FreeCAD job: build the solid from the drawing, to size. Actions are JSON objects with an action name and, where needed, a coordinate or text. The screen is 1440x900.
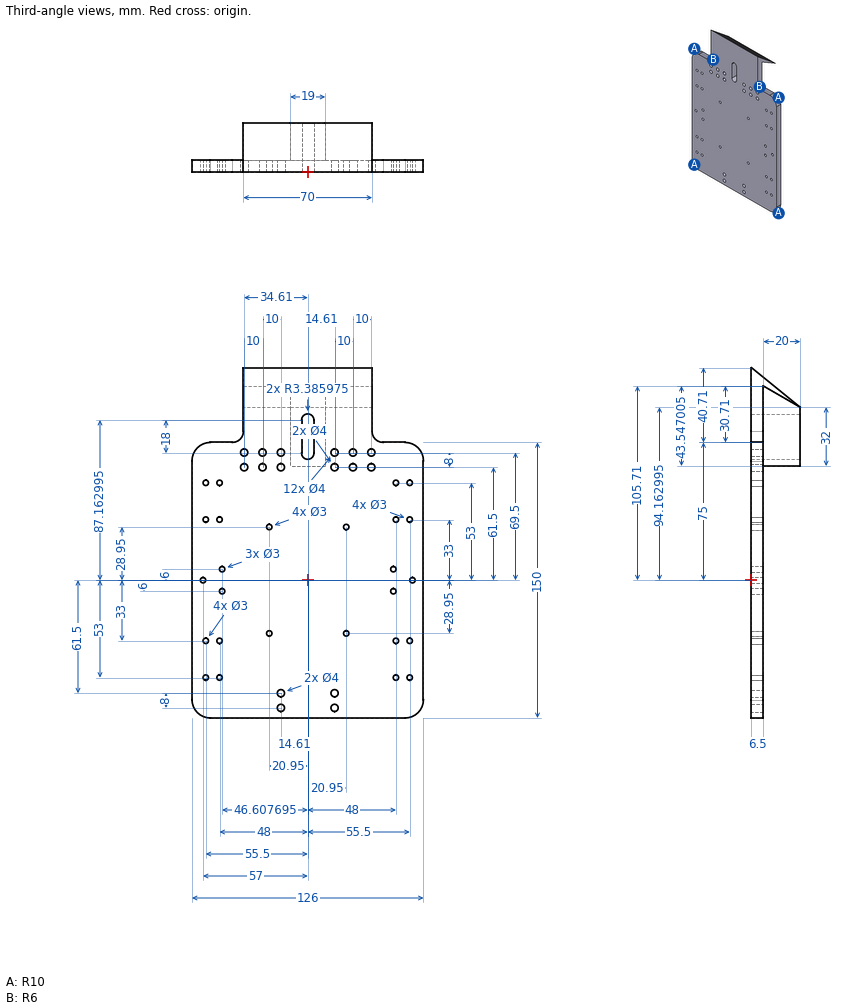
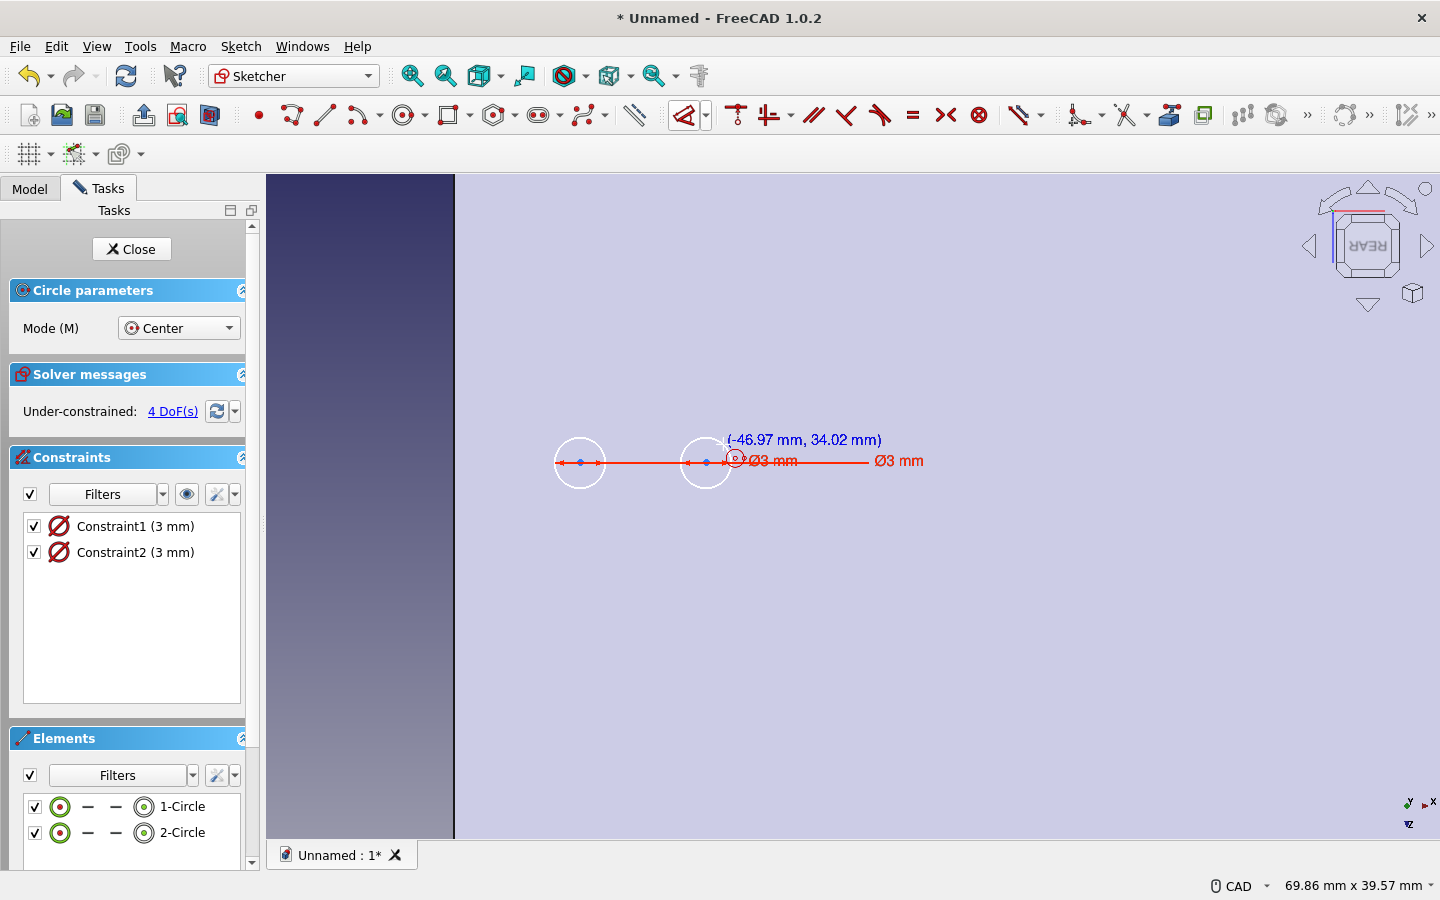
{"action": "scroll", "coordinate": [581, 464], "scroll_direction": "down", "scroll_amount": 4}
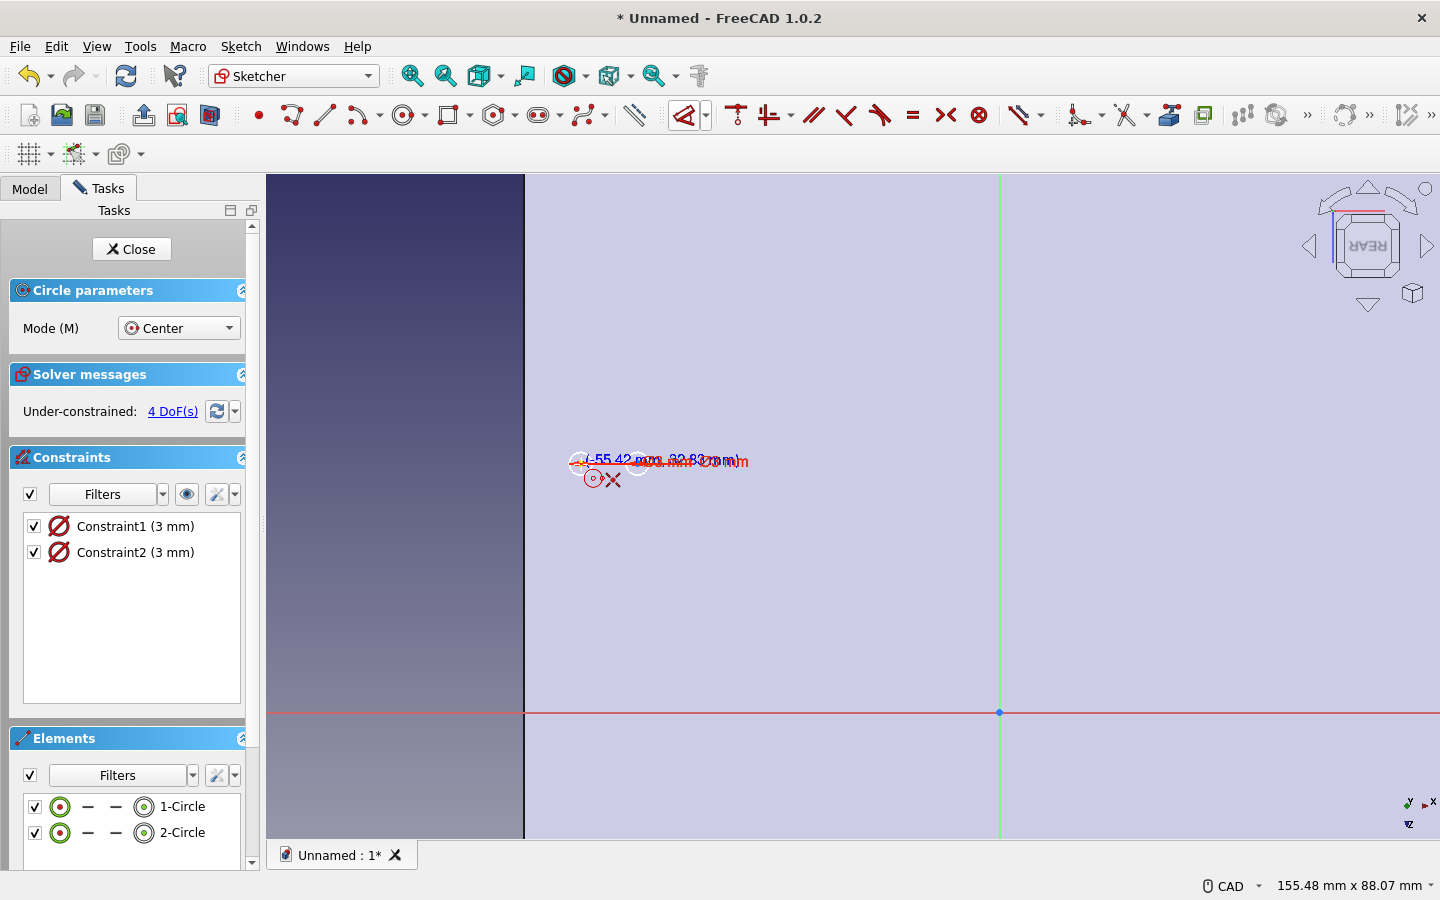
{"action": "scroll", "coordinate": [637, 312], "scroll_direction": "up", "scroll_amount": 4}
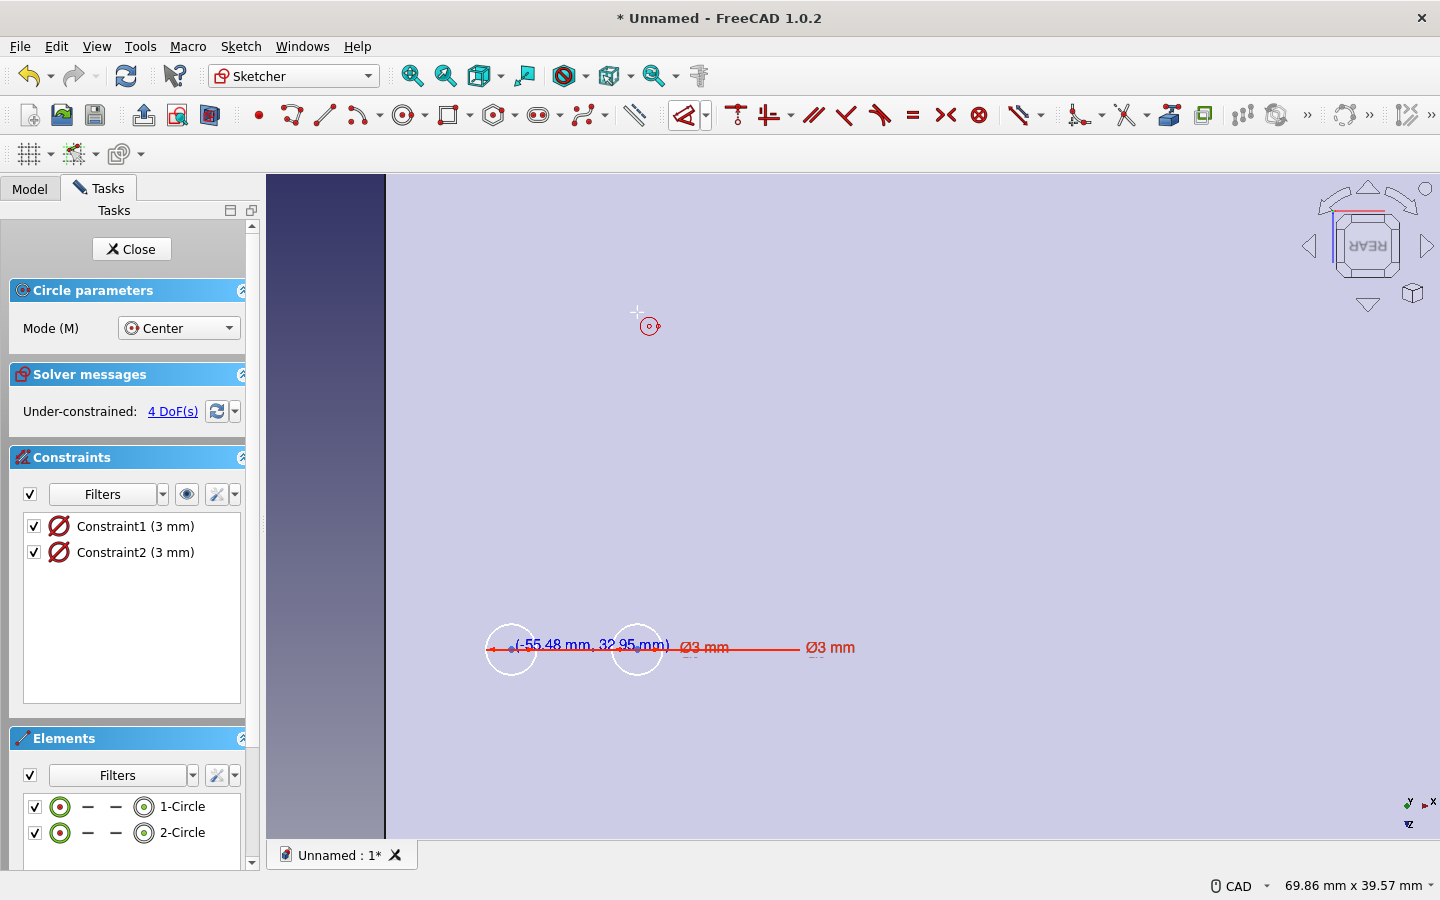
{"action": "left_click", "coordinate": [637, 313]}
{"action": "mouse_move", "coordinate": [655, 295]}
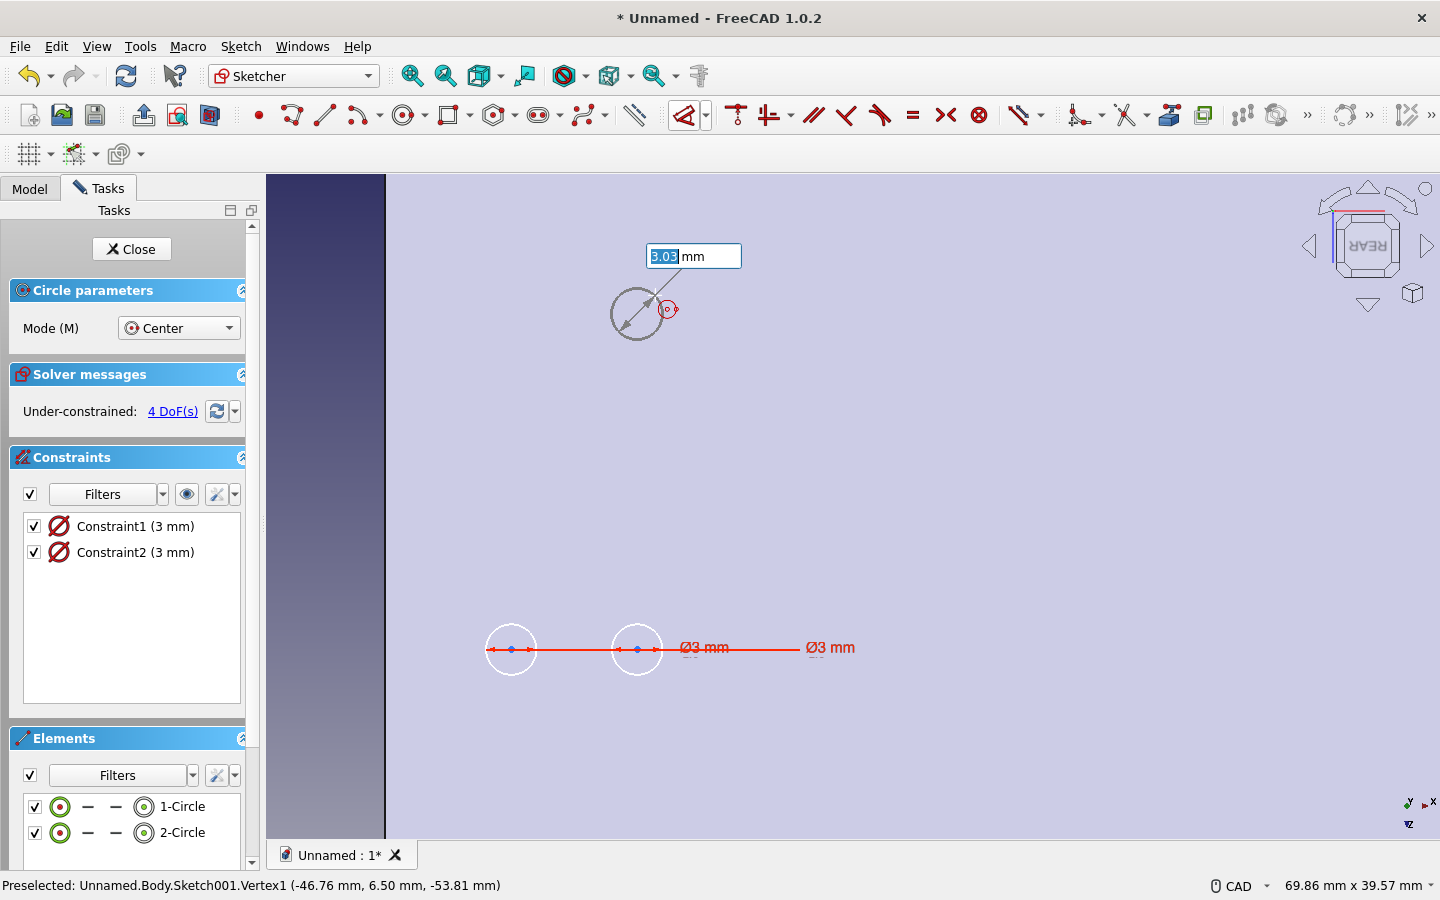
{"action": "type", "text": "3"}
{"action": "key", "text": "Return"}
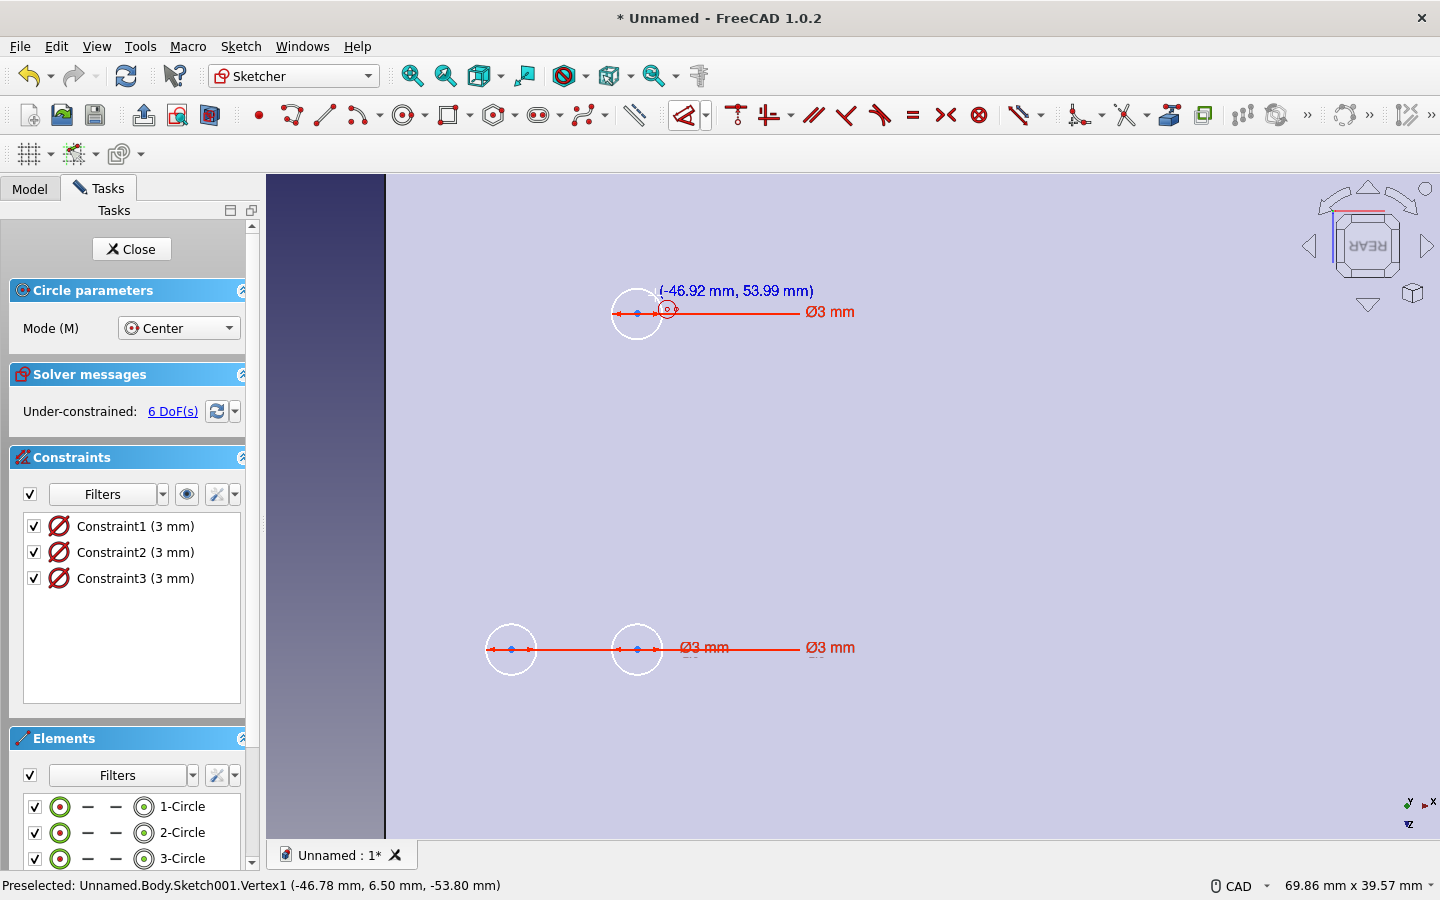
{"action": "left_click", "coordinate": [511, 313]}
{"action": "mouse_move", "coordinate": [529, 295]}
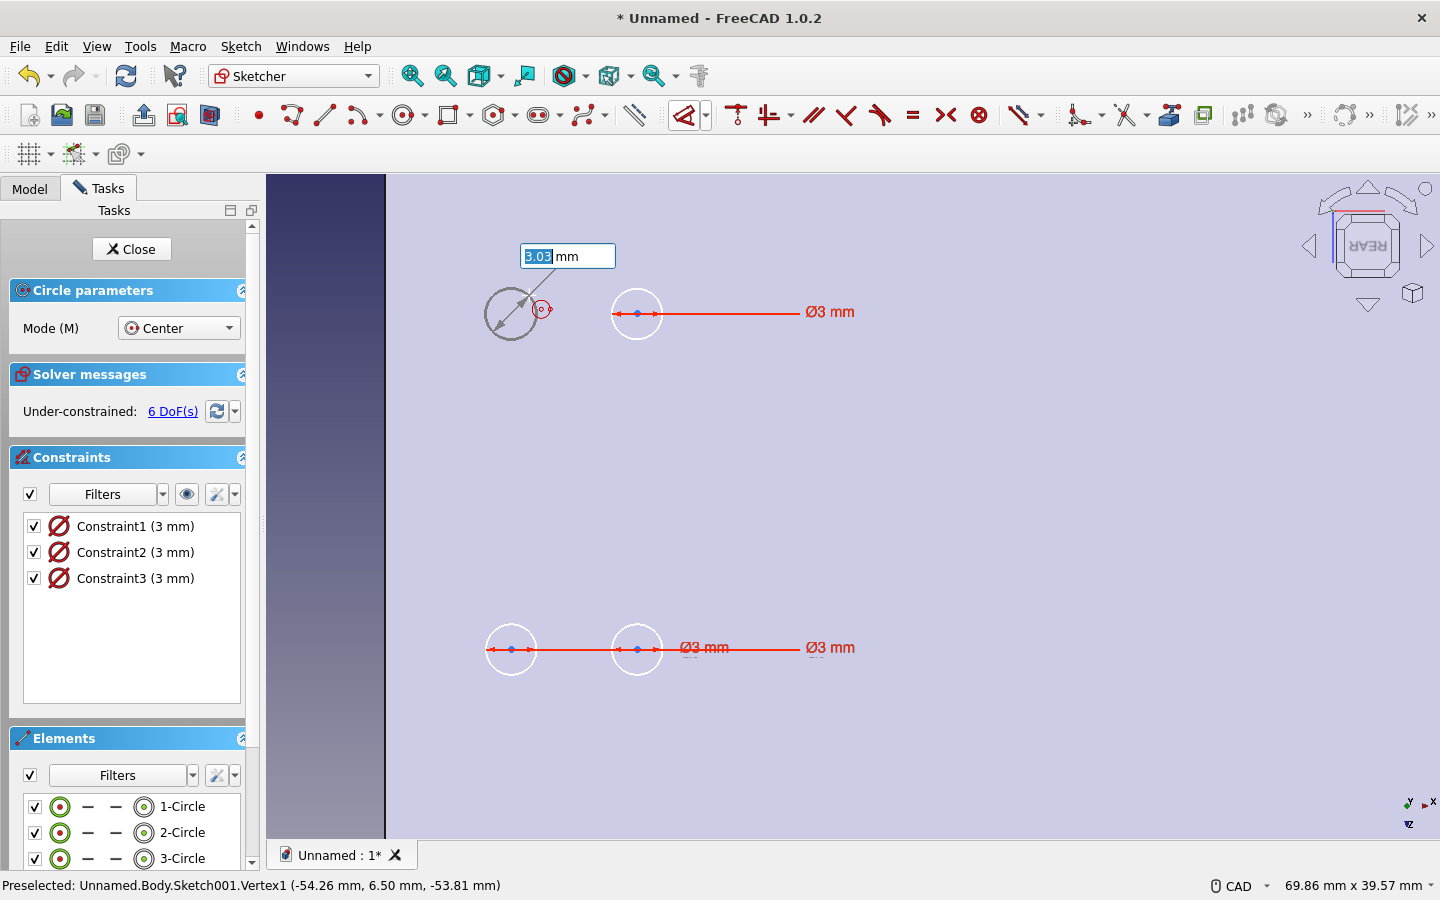
{"action": "type", "text": "3"}
{"action": "key", "text": "Return"}
{"action": "key", "text": "Escape"}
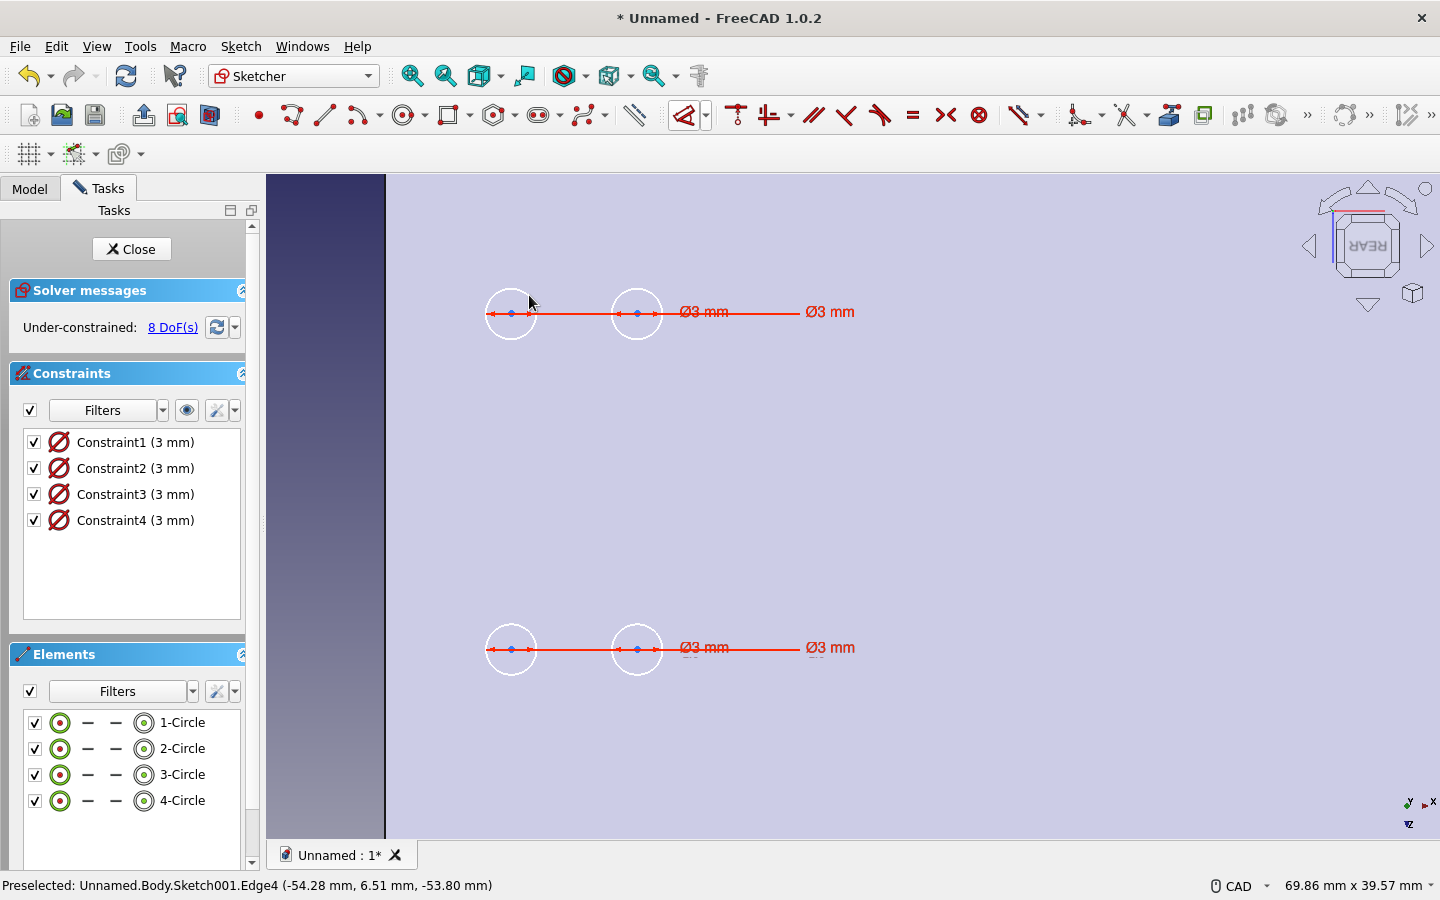
{"action": "left_click", "coordinate": [511, 650]}